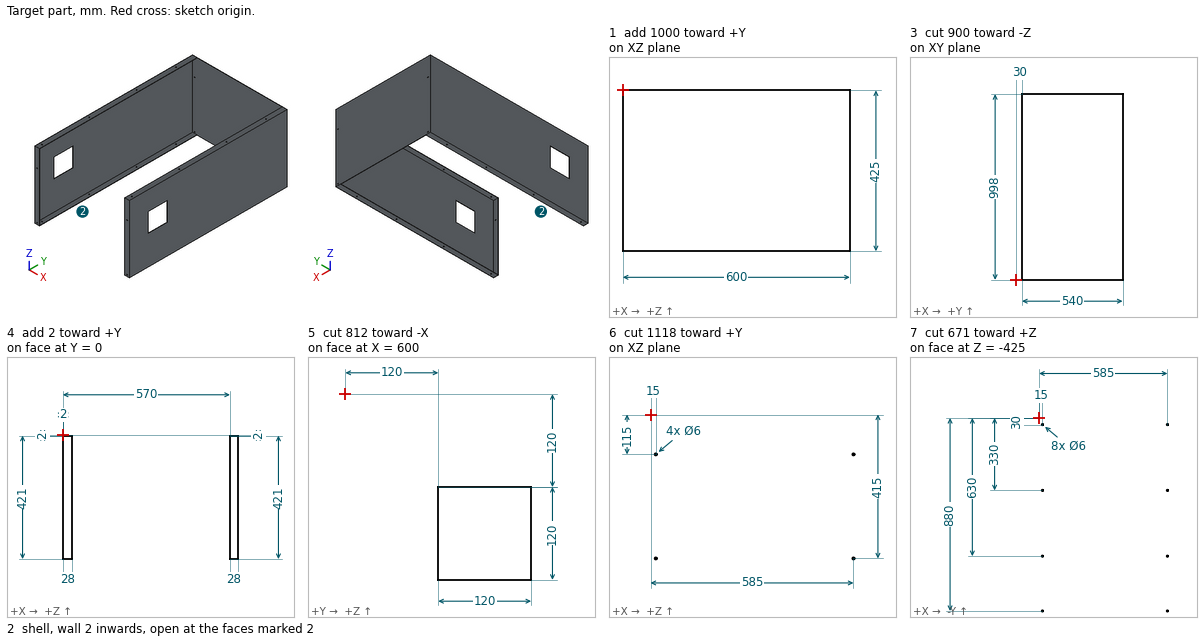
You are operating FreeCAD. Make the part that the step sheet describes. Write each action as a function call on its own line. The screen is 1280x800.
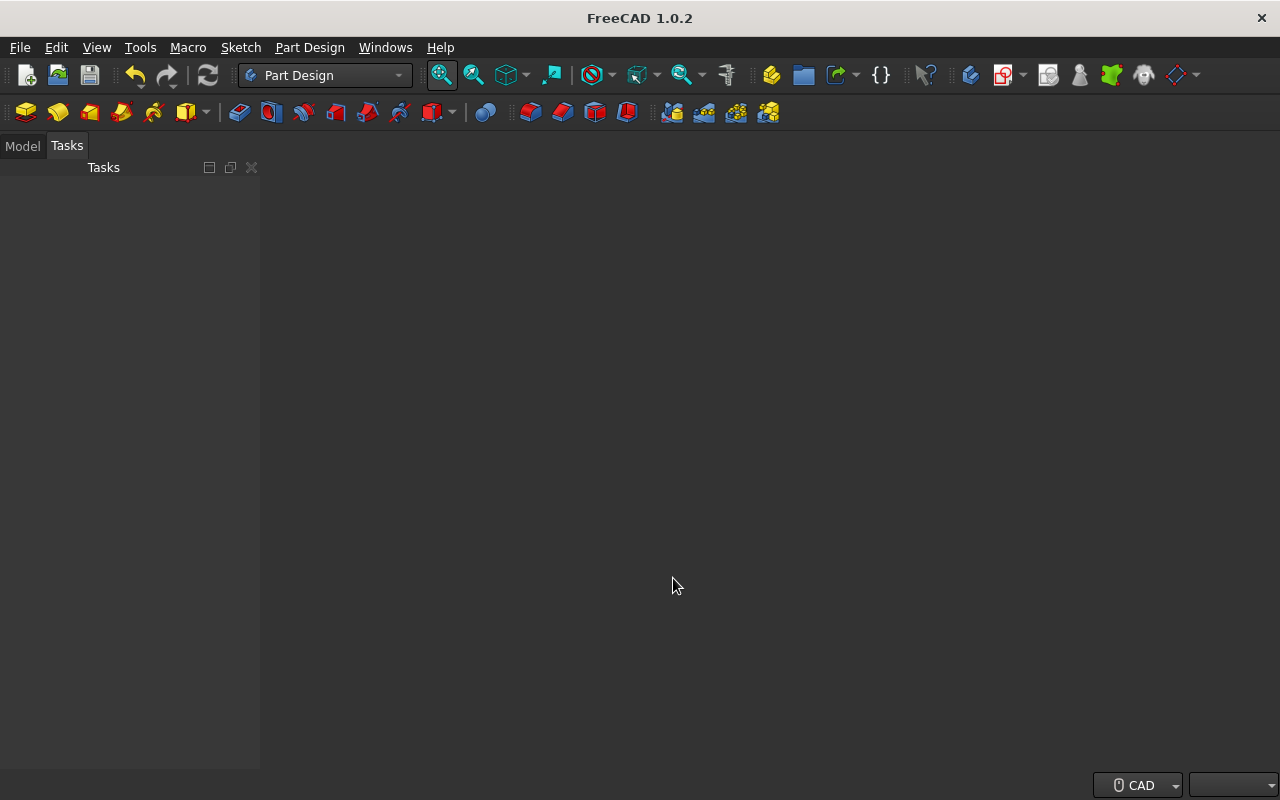
click(26, 76)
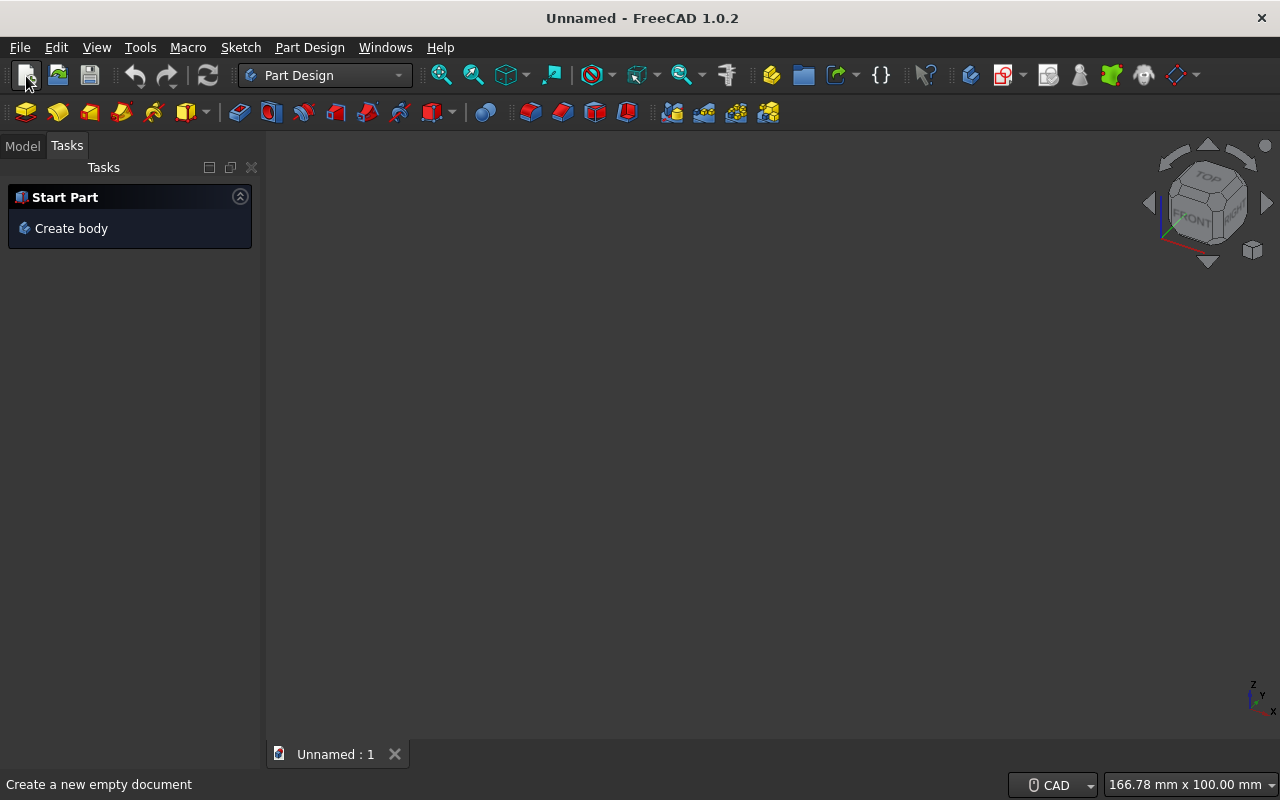
click(1004, 76)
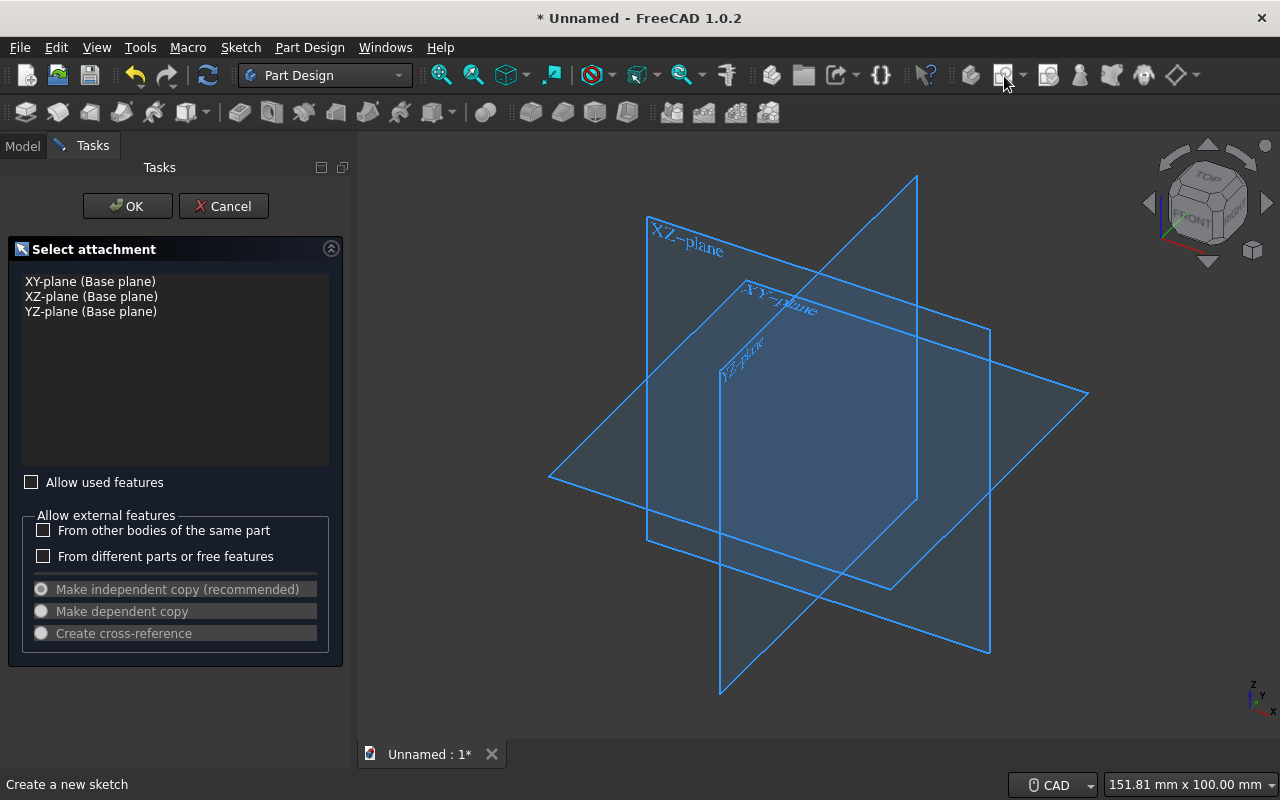
click(82, 296)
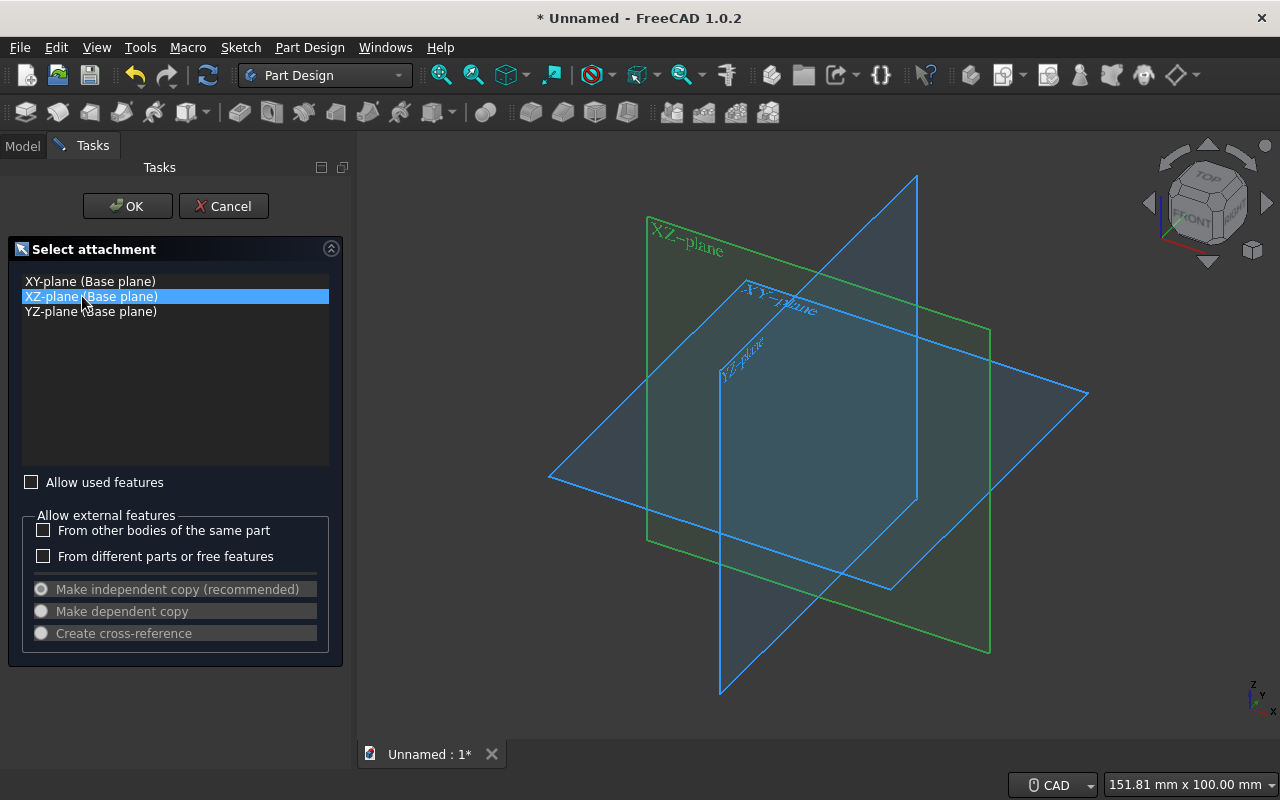
click(128, 206)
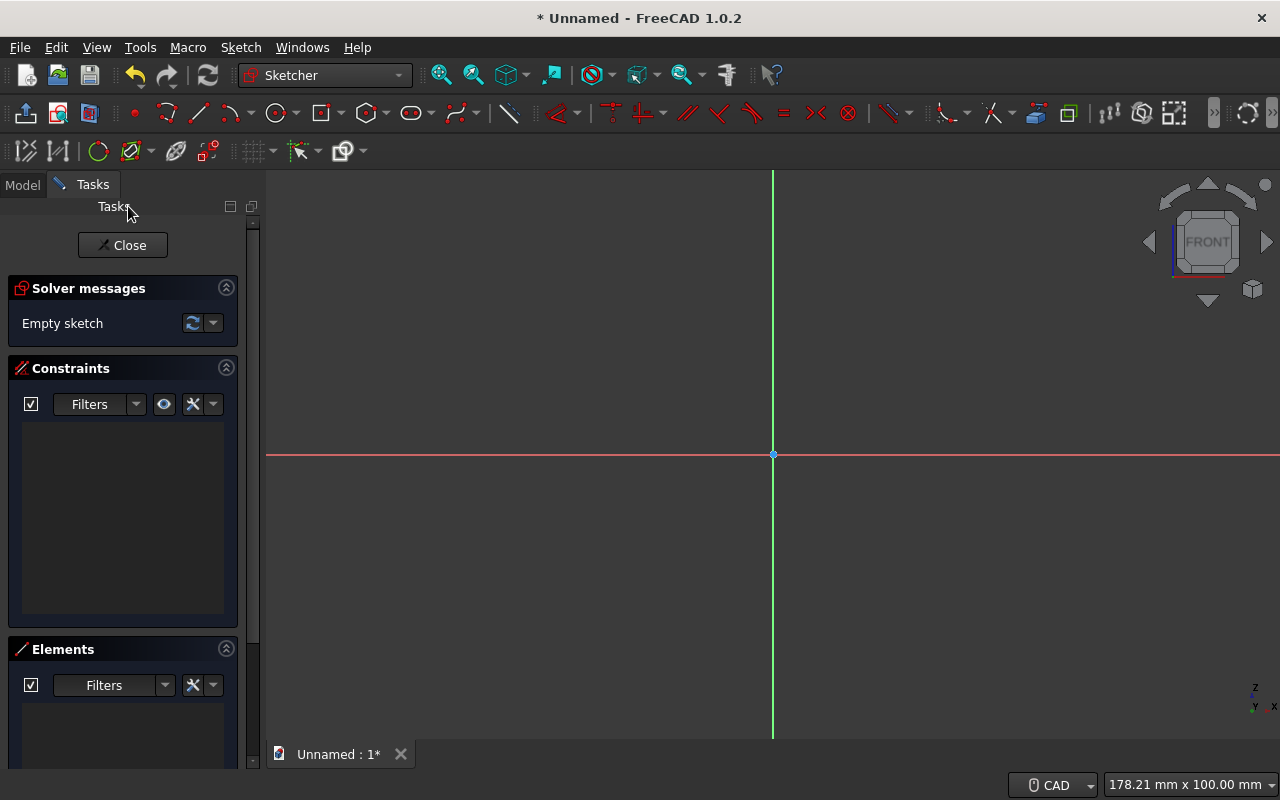
scroll(353, 215, down, 9)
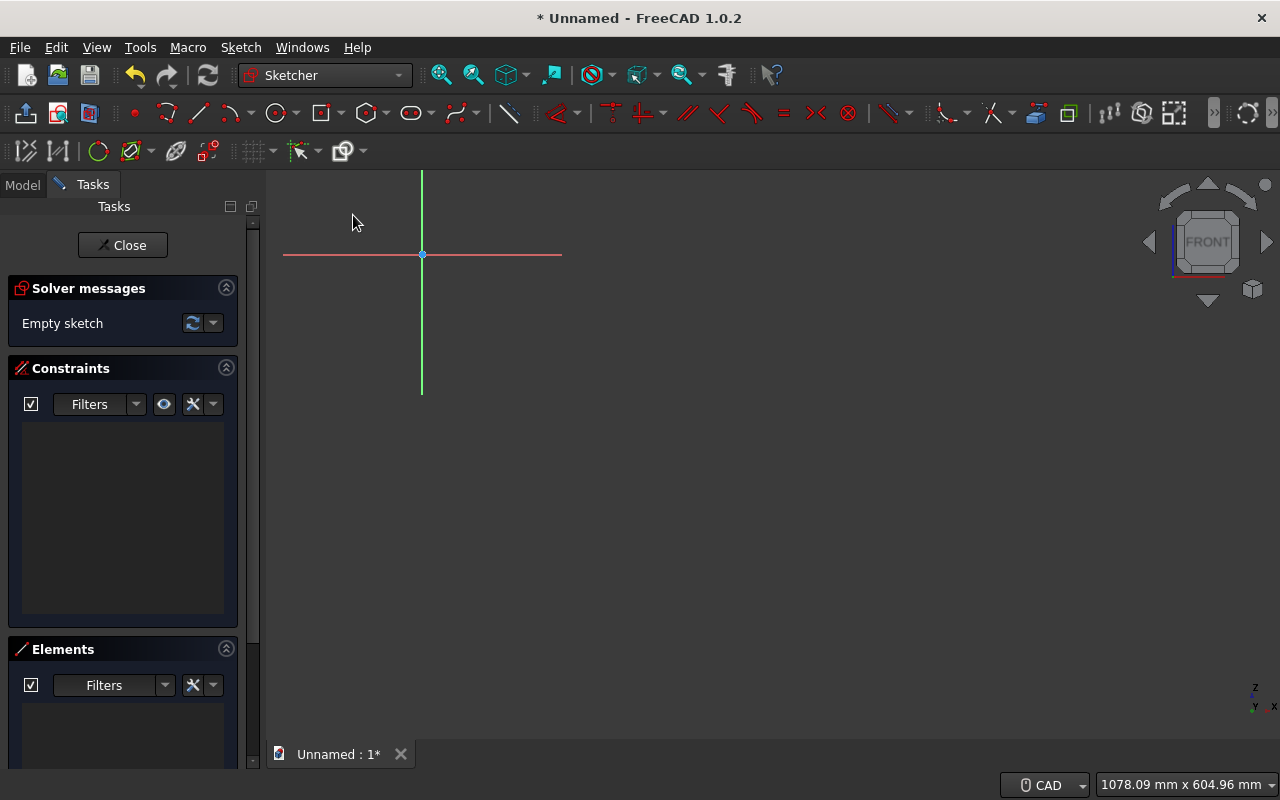
click(344, 114)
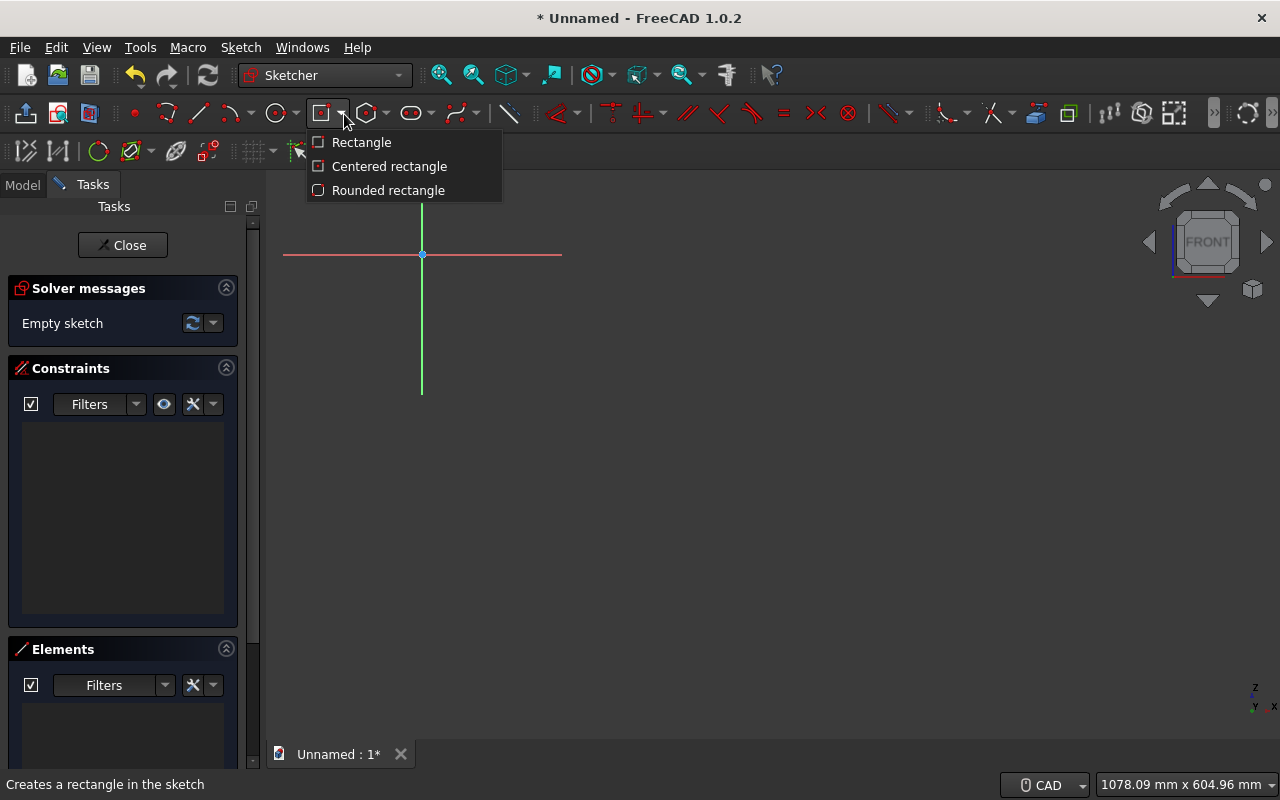
click(404, 142)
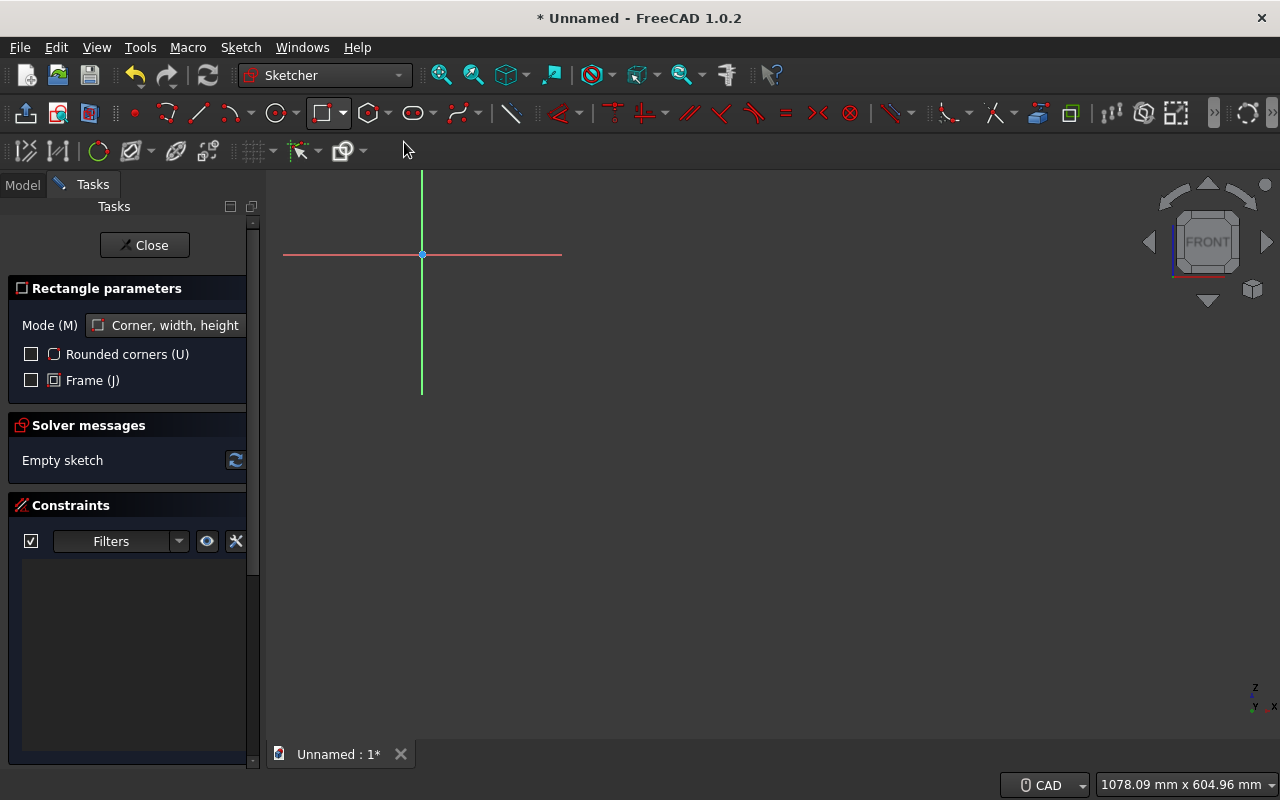
click(422, 255)
move(987, 654)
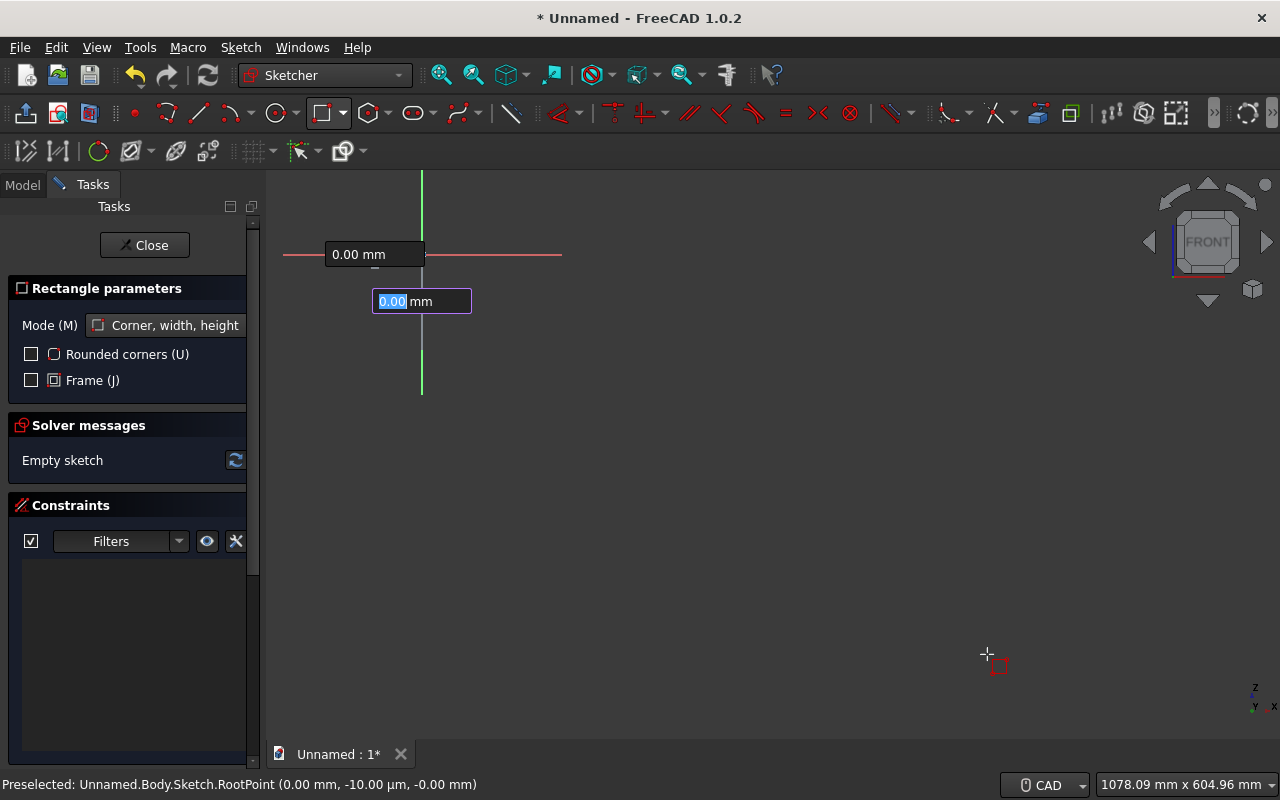
text(600)
key(Tab)
text(425)
key(Return)
key(Escape)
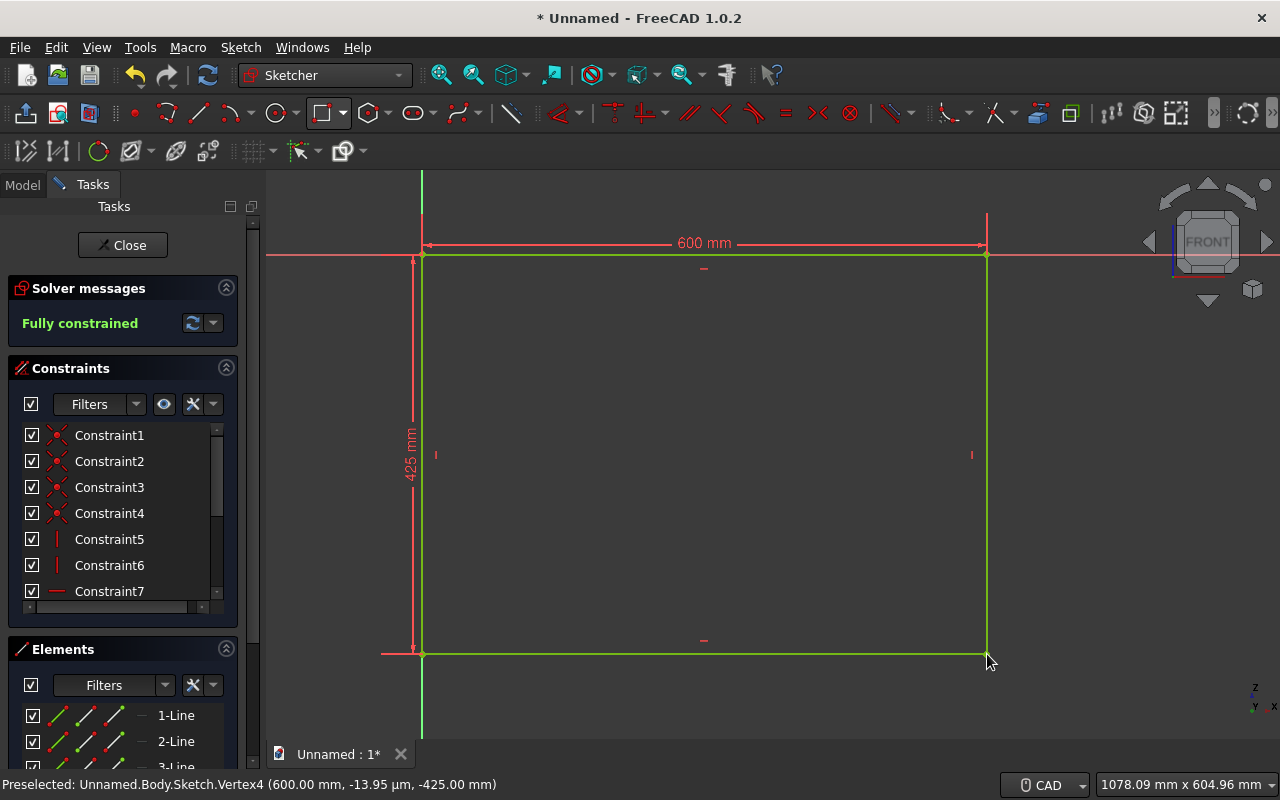
click(123, 245)